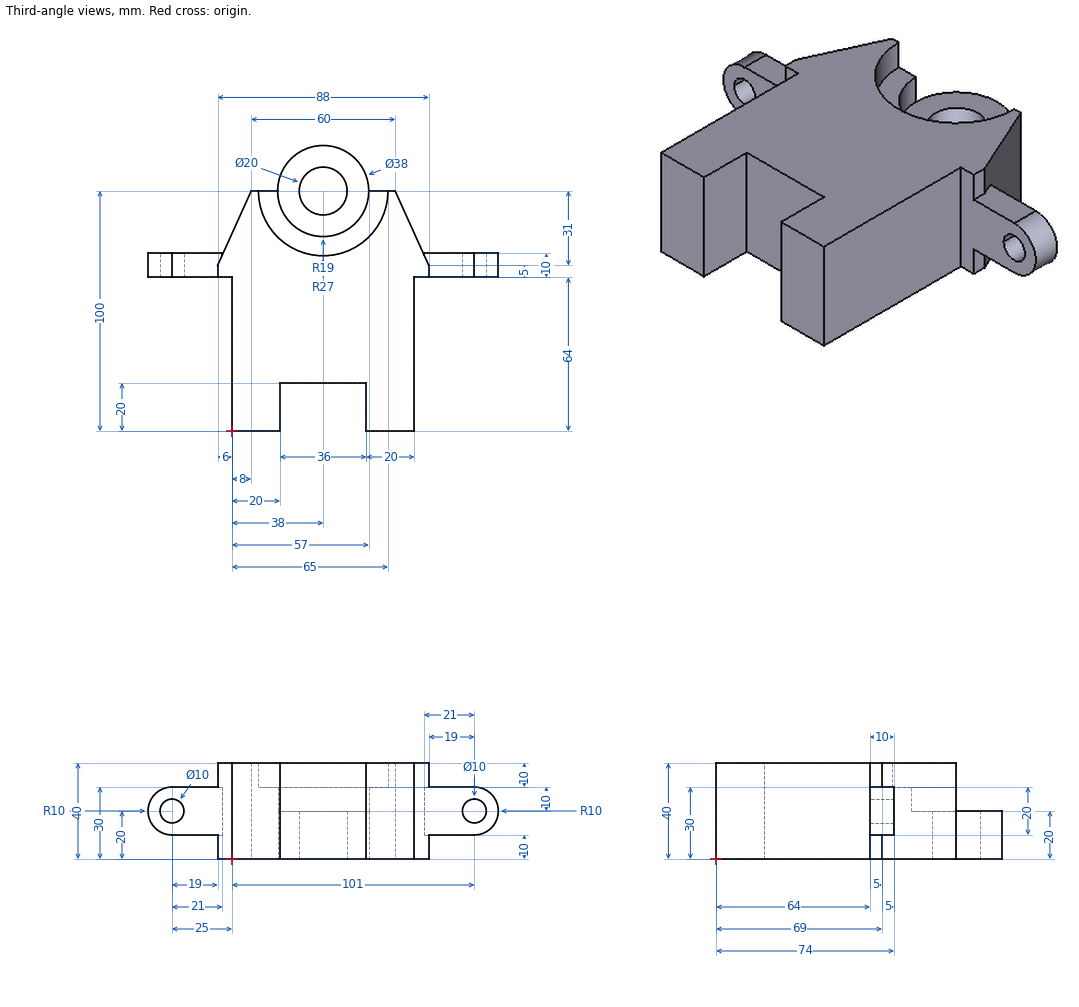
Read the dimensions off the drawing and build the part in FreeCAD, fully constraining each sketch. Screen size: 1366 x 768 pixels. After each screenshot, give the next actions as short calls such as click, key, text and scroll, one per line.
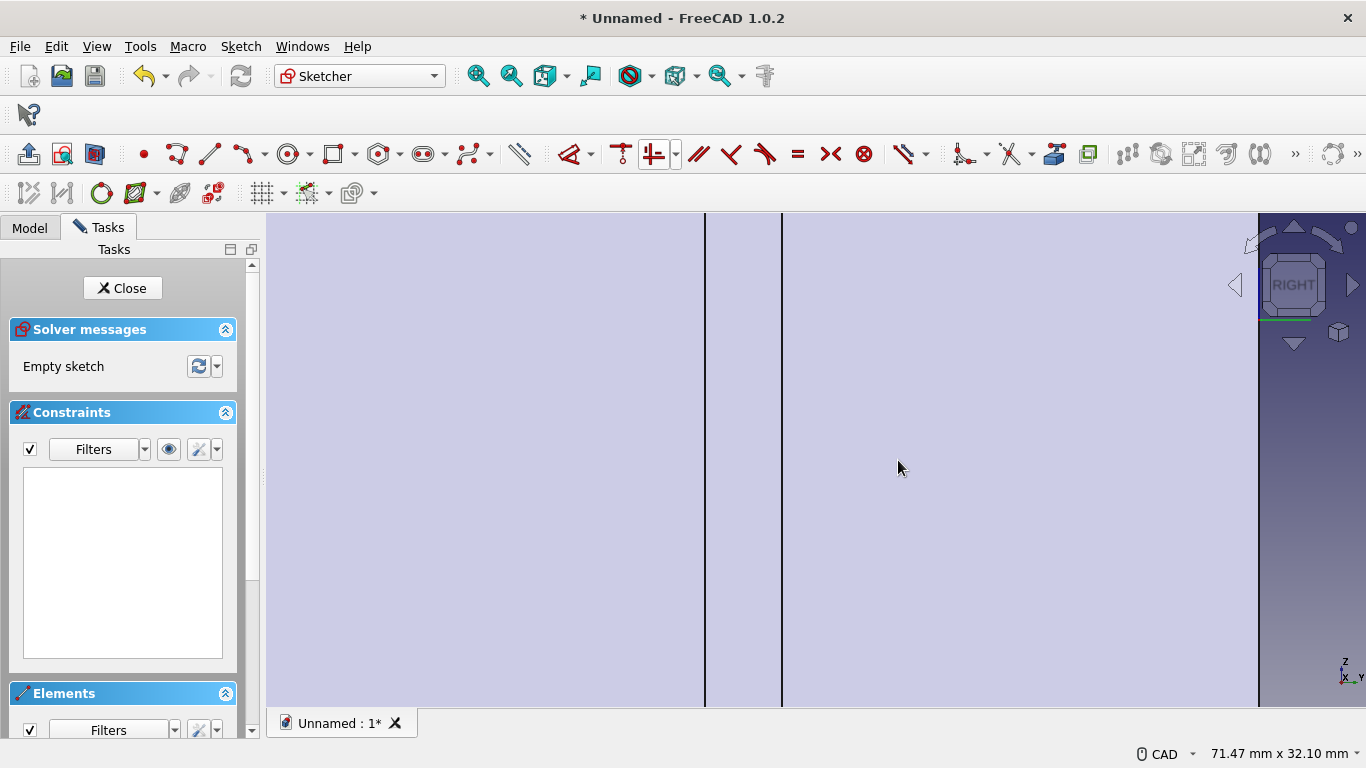
click(332, 154)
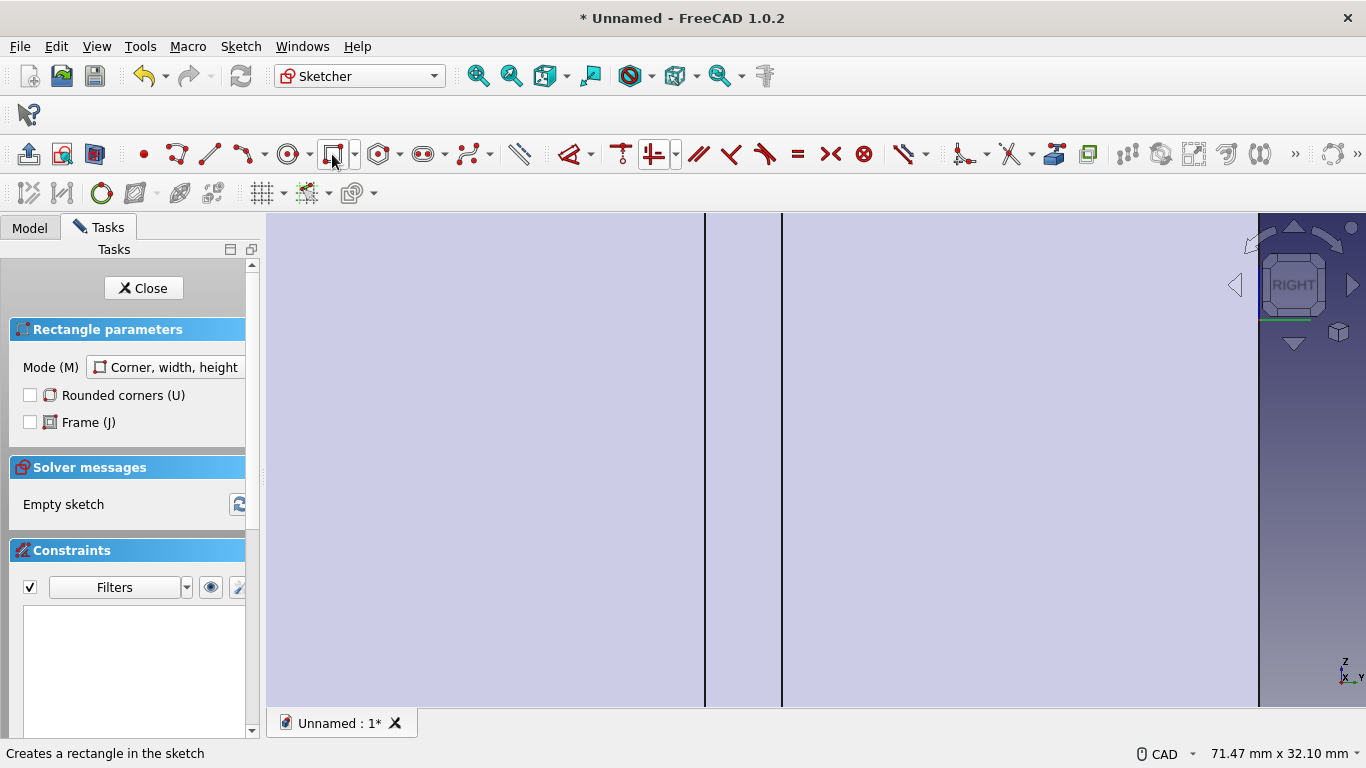
click(705, 304)
click(782, 612)
key(Escape)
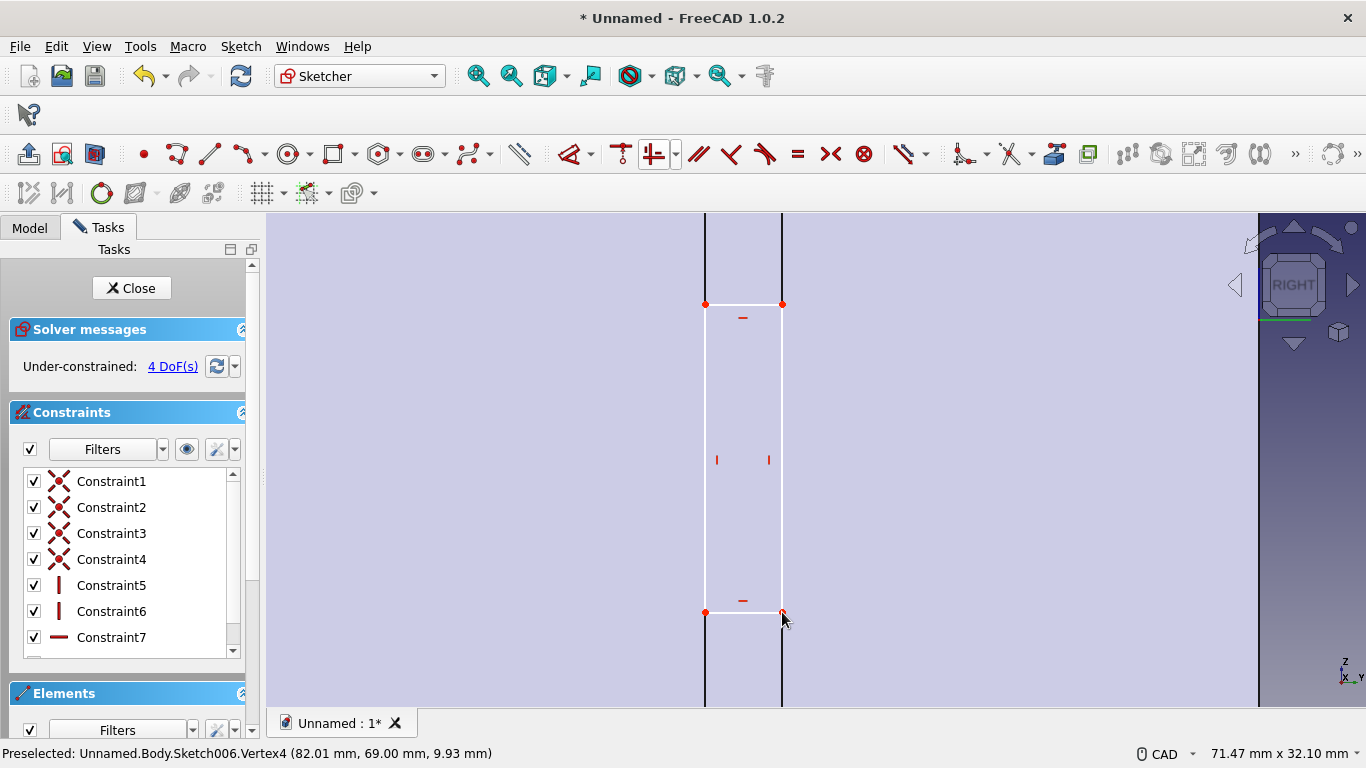
click(568, 154)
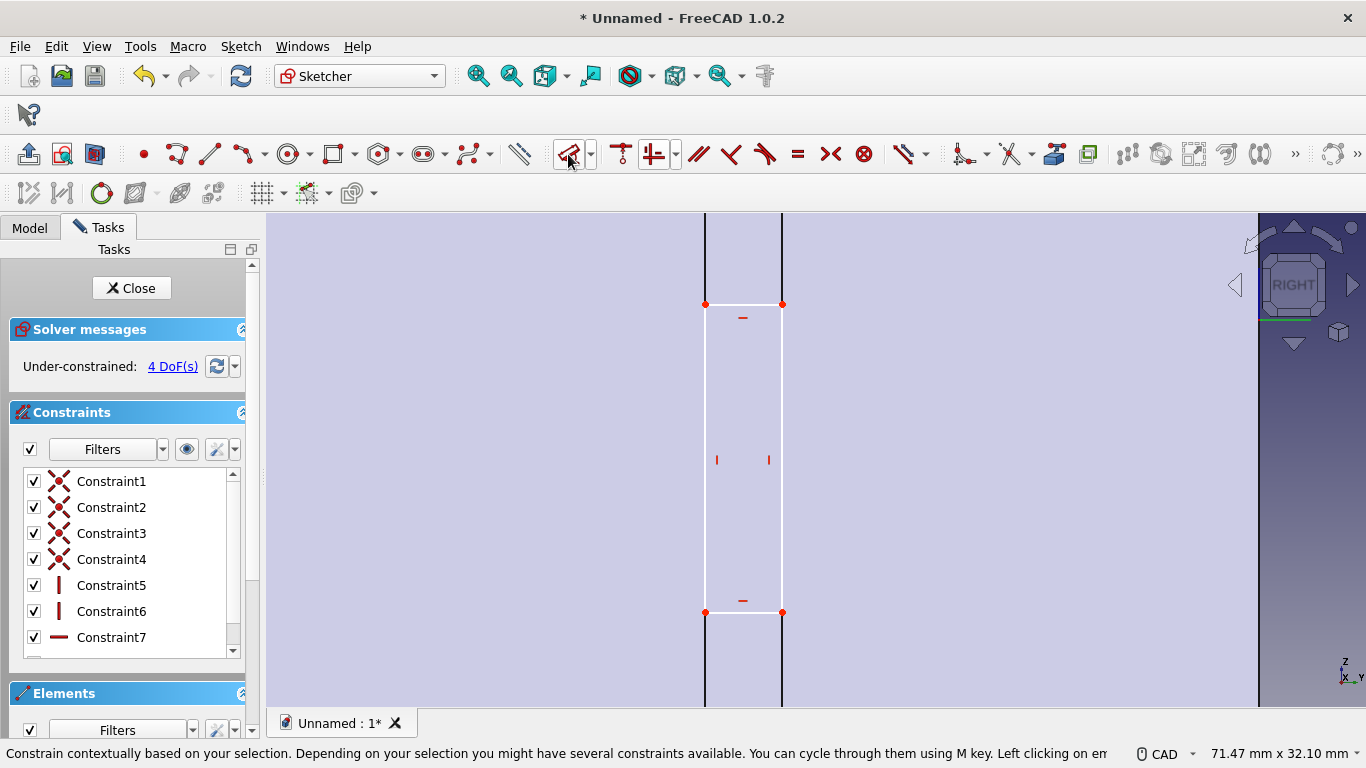
click(728, 613)
click(744, 647)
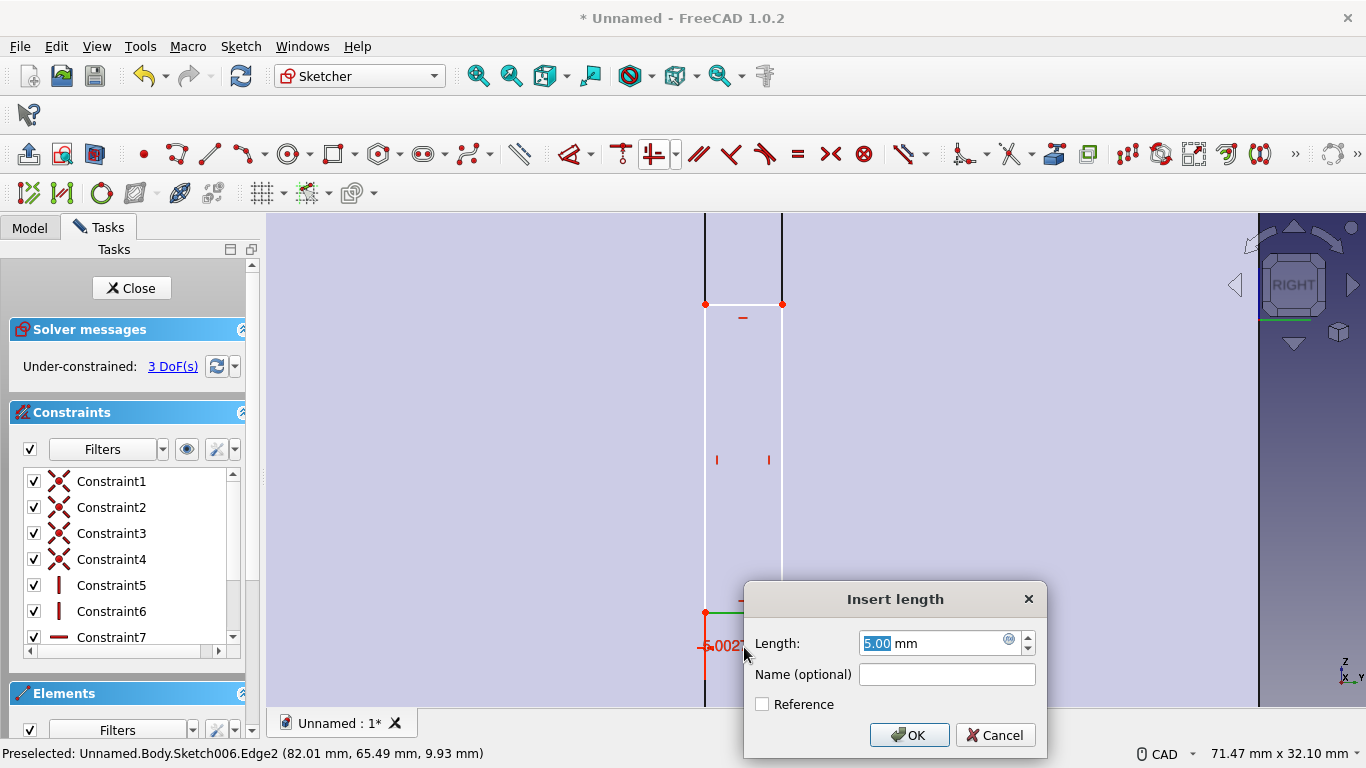
text(5)
key(Return)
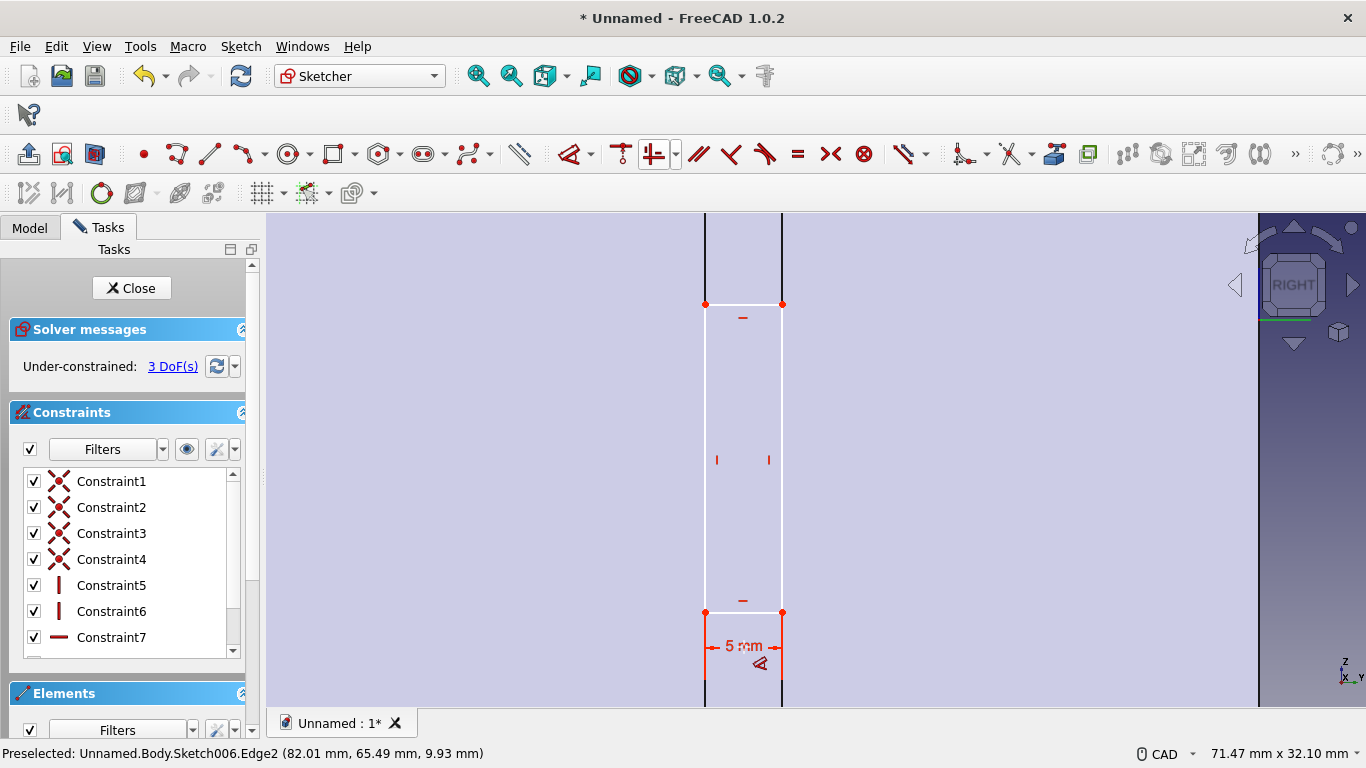
click(705, 397)
click(671, 459)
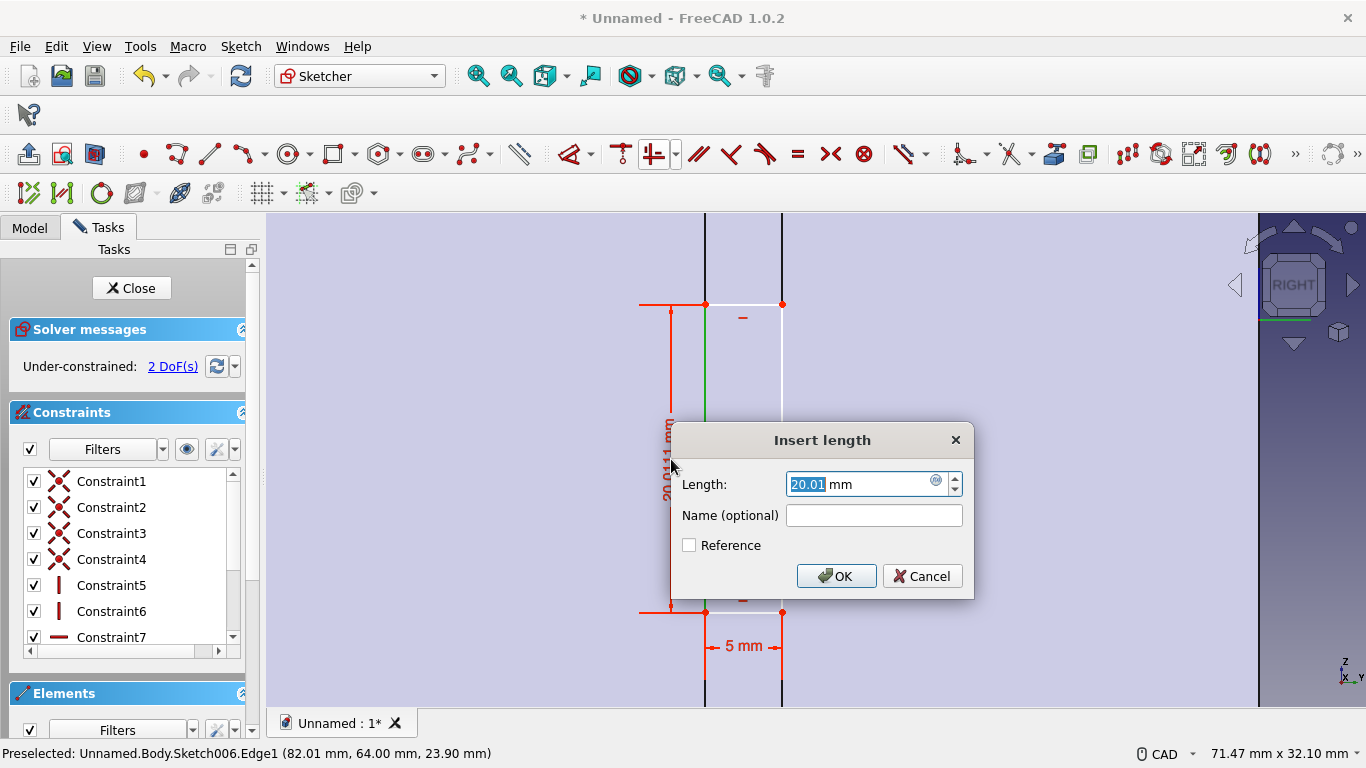
text(20)
key(Return)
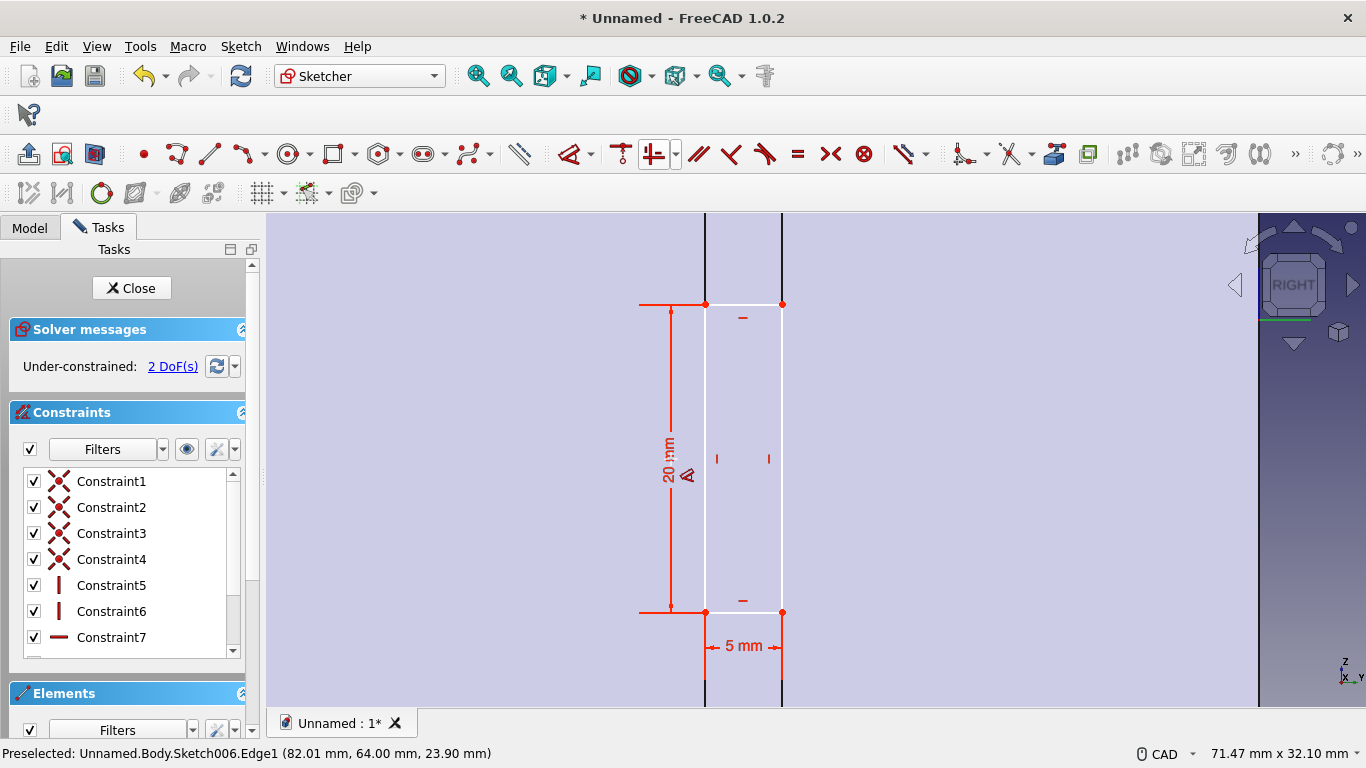
click(705, 305)
click(500, 271)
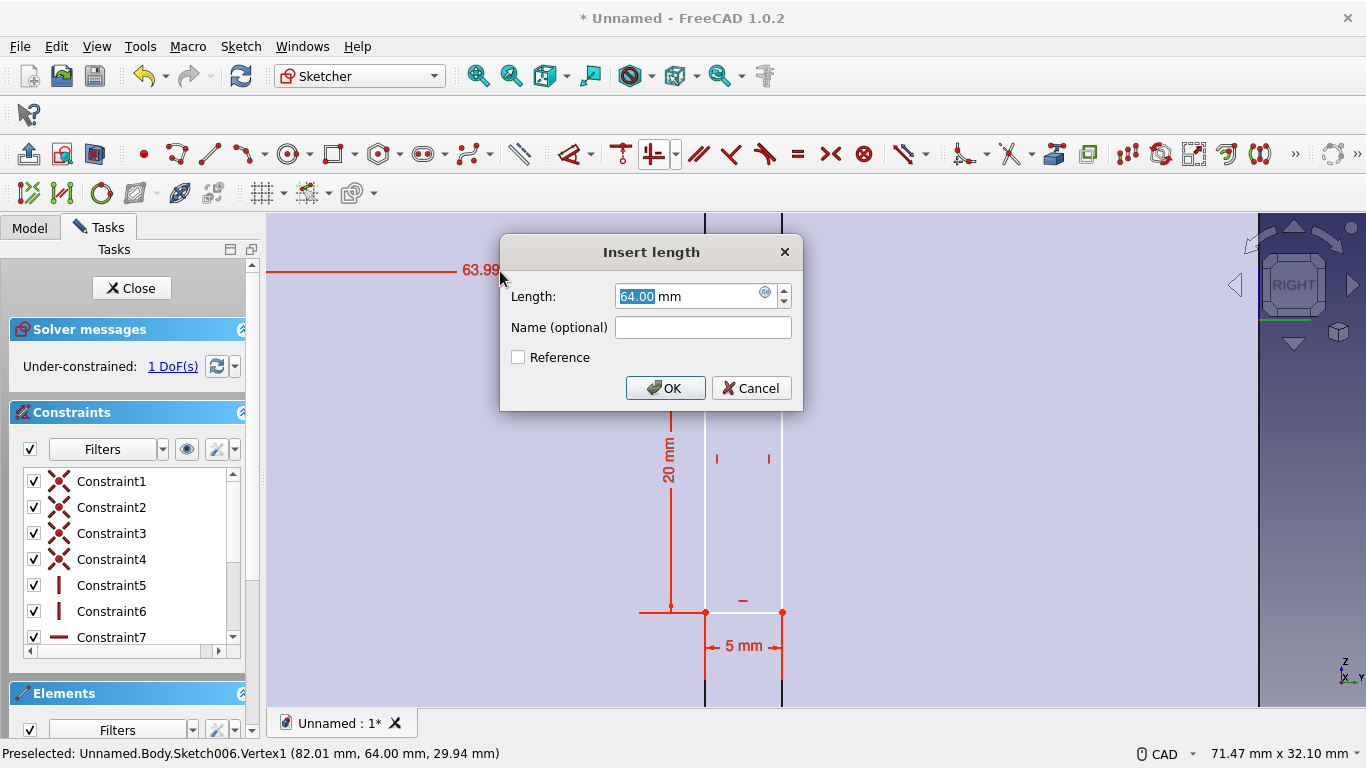
text(64)
key(Return)